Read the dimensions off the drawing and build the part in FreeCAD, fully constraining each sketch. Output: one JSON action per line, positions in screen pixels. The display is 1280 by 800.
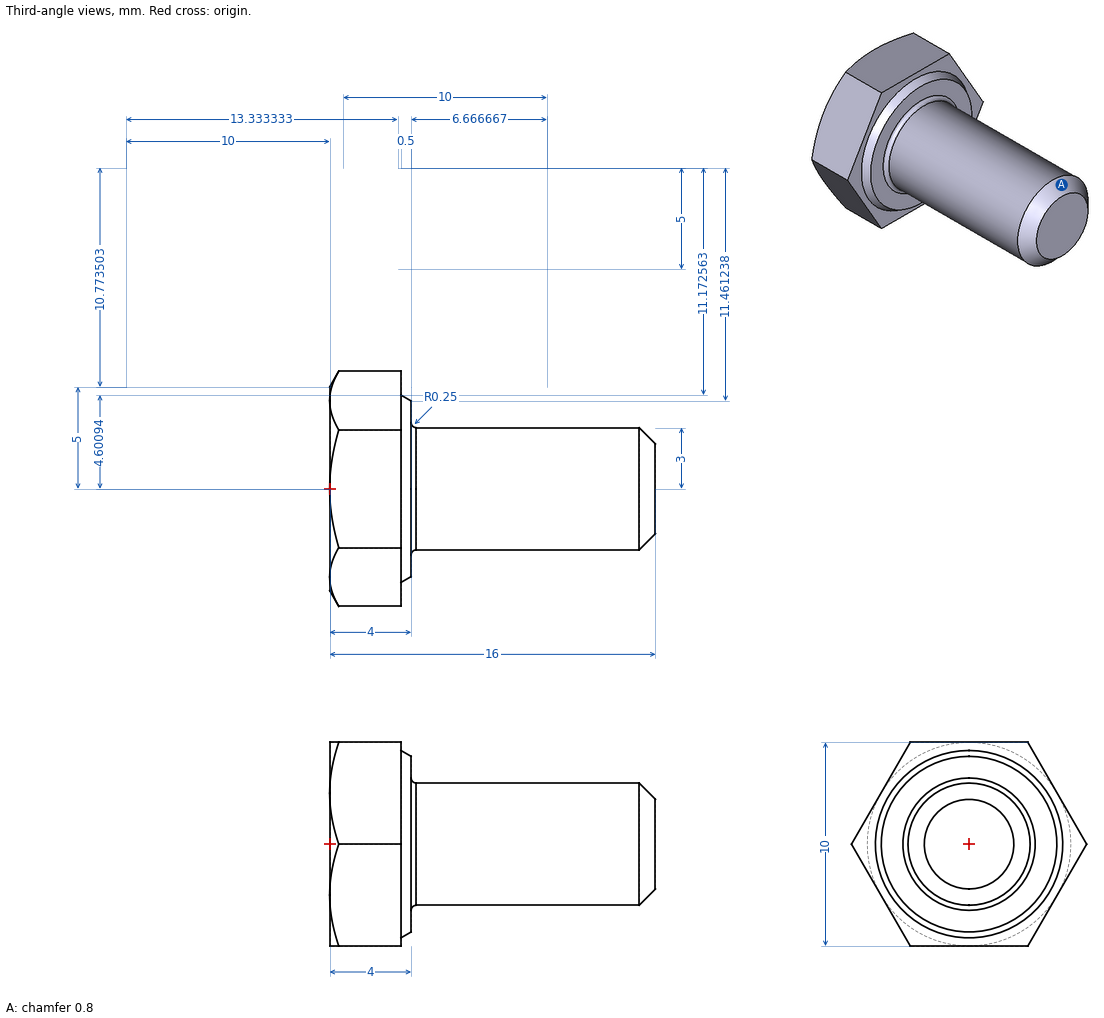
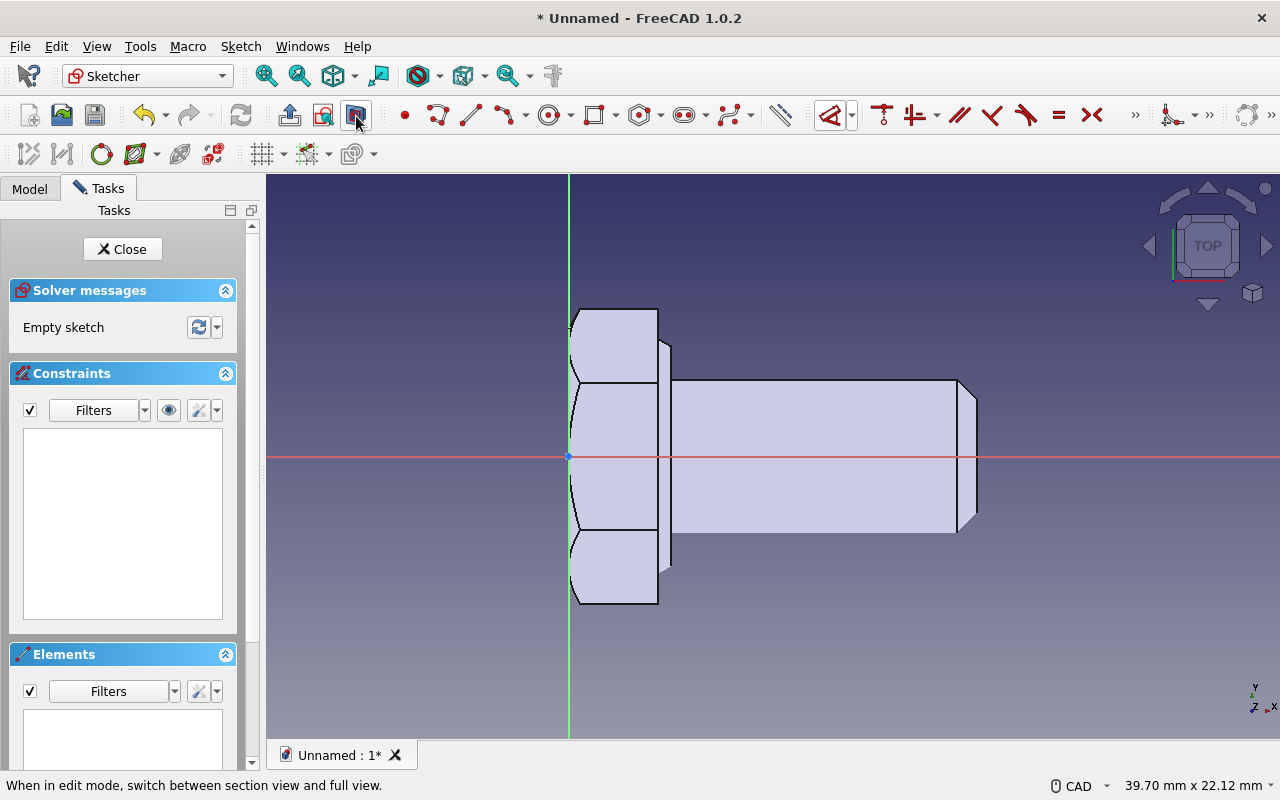
{"action": "scroll", "coordinate": [672, 373], "scroll_direction": "up", "scroll_amount": 15}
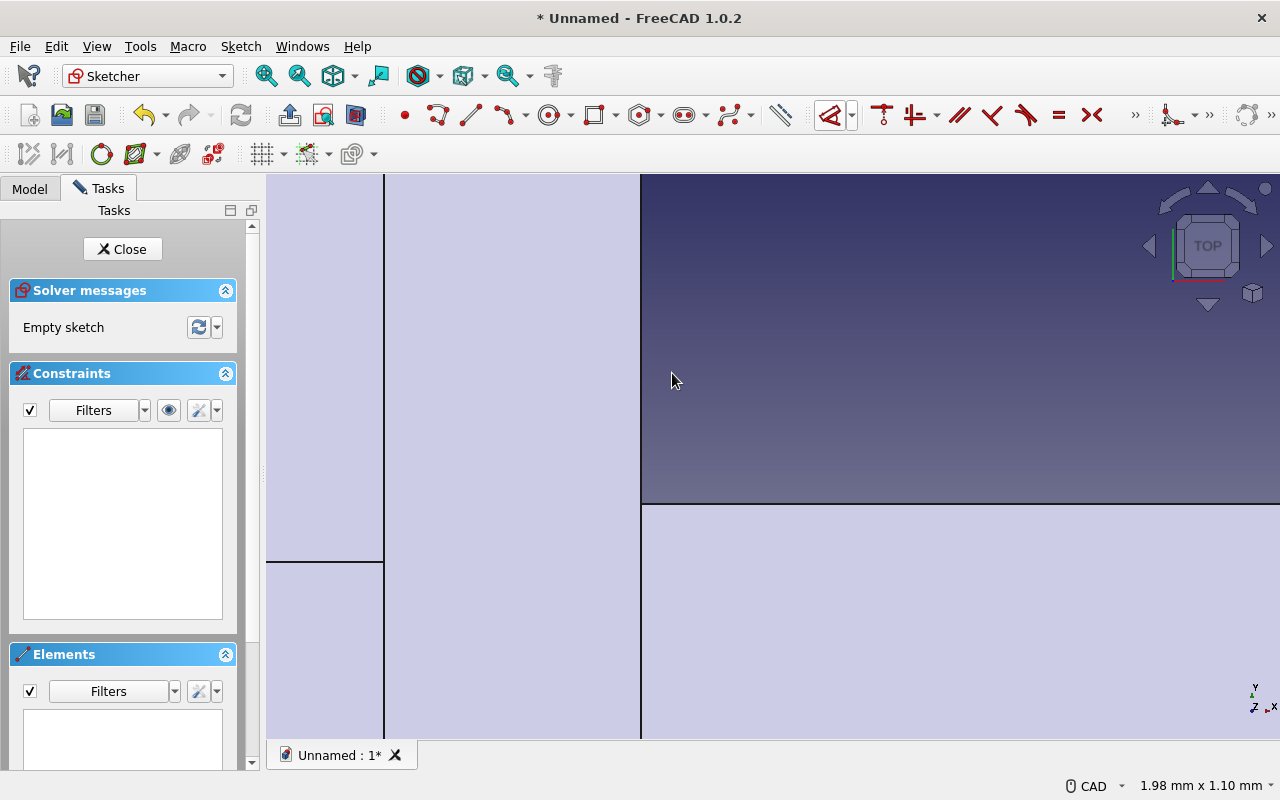
{"action": "scroll", "coordinate": [705, 431], "scroll_direction": "up", "scroll_amount": 5}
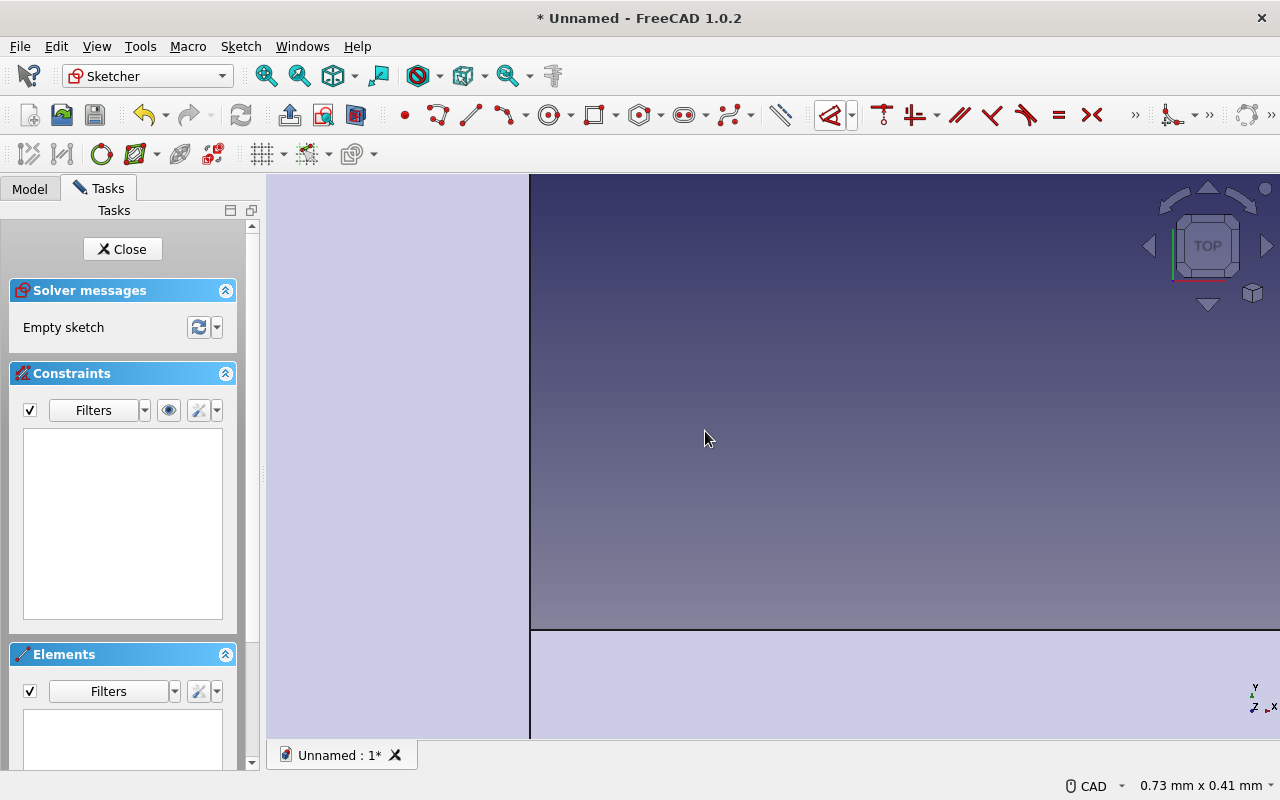
{"action": "left_click", "coordinate": [438, 116]}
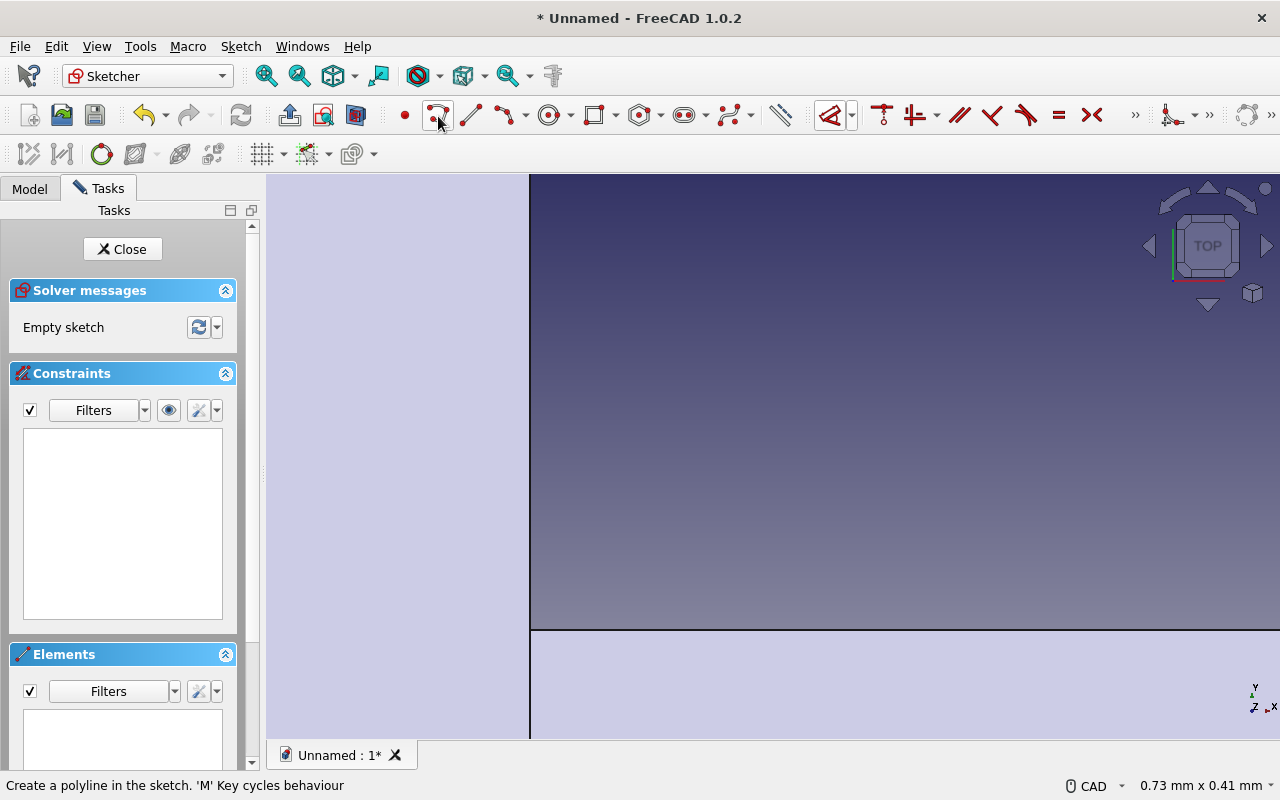
{"action": "left_click", "coordinate": [530, 281]}
{"action": "left_click", "coordinate": [530, 630]}
{"action": "left_click", "coordinate": [879, 630]}
{"action": "right_click", "coordinate": [879, 630]}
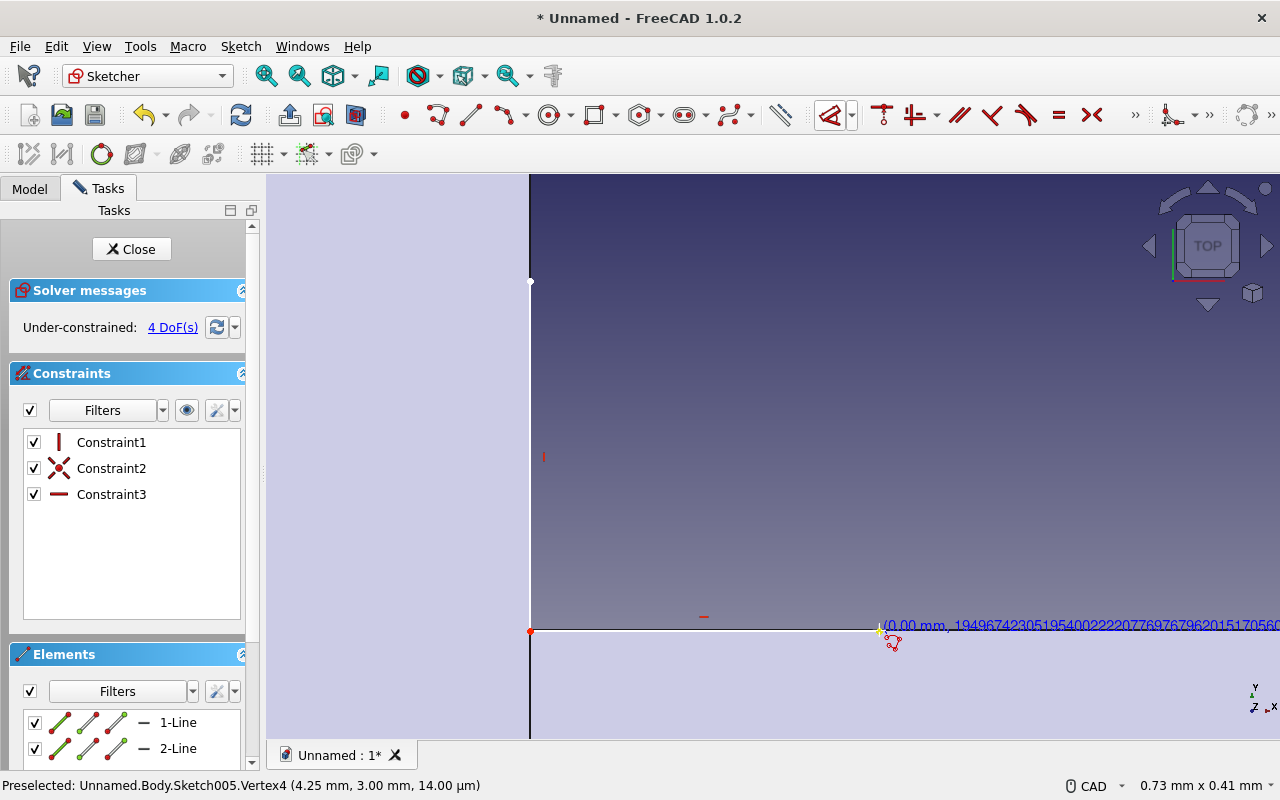
{"action": "left_click", "coordinate": [504, 116]}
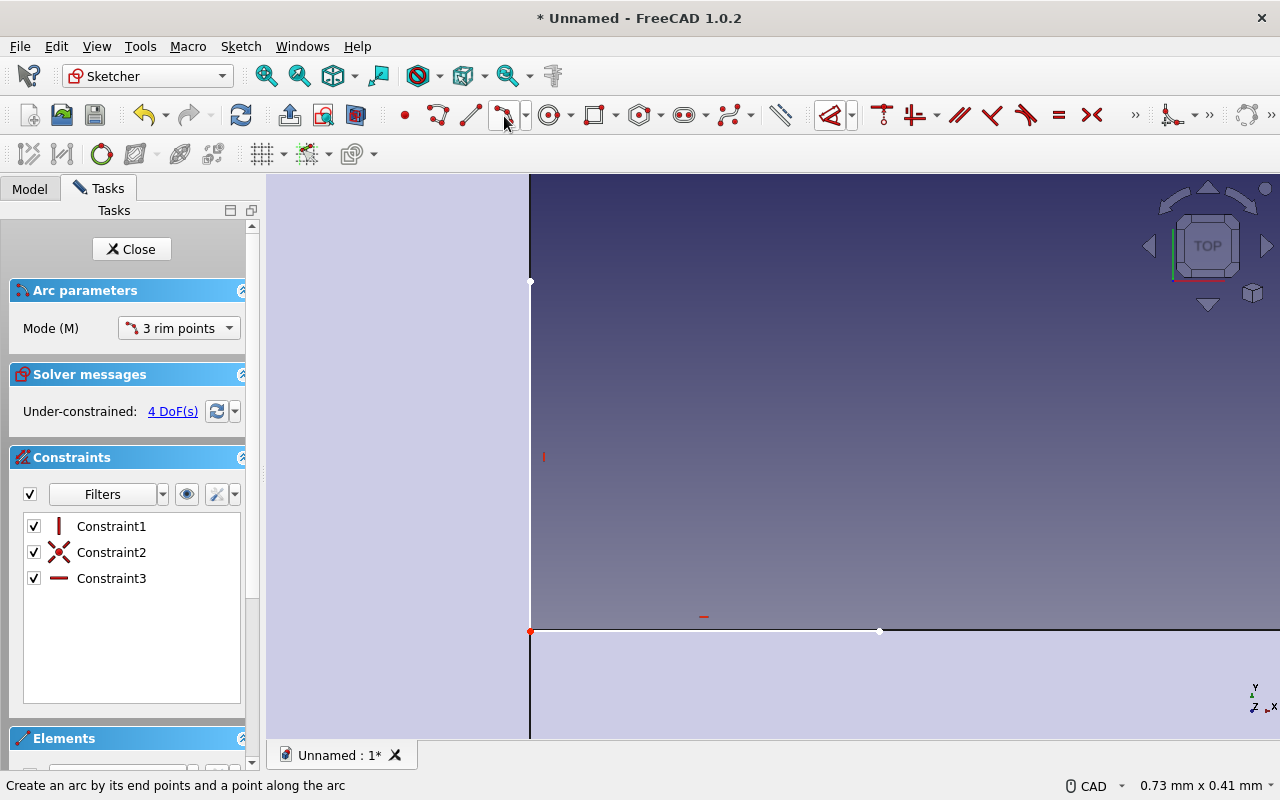
{"action": "left_click", "coordinate": [879, 631]}
{"action": "left_click", "coordinate": [530, 282]}
{"action": "left_click", "coordinate": [632, 528]}
{"action": "key", "text": "Escape"}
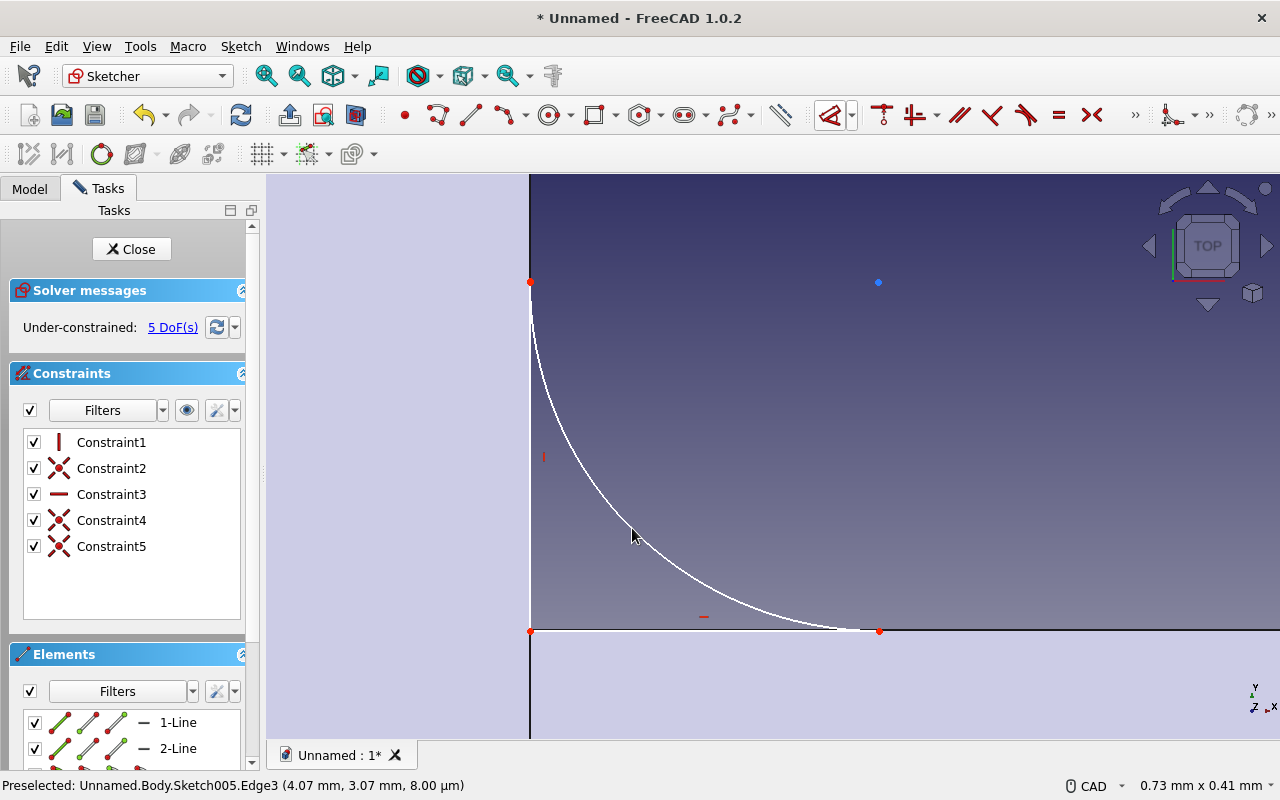
{"action": "left_click", "coordinate": [530, 387]}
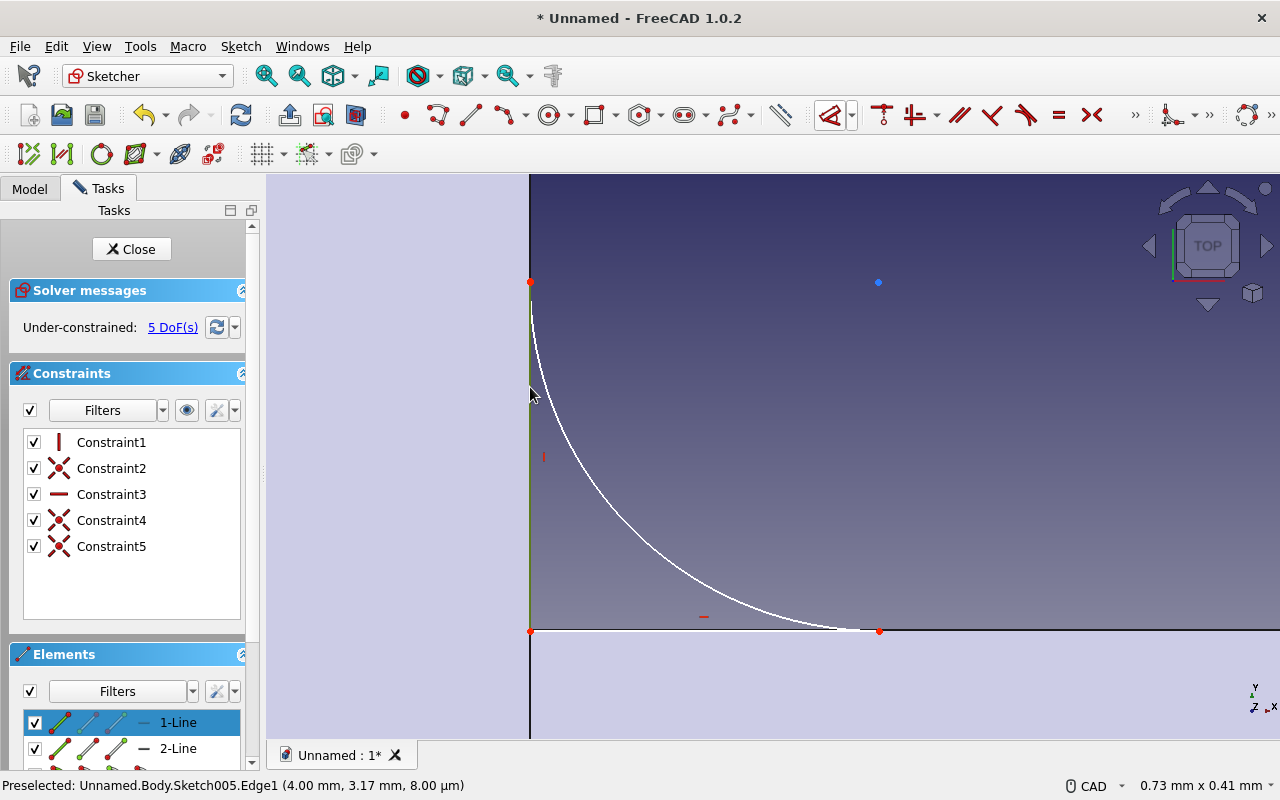
{"action": "left_click", "coordinate": [568, 441]}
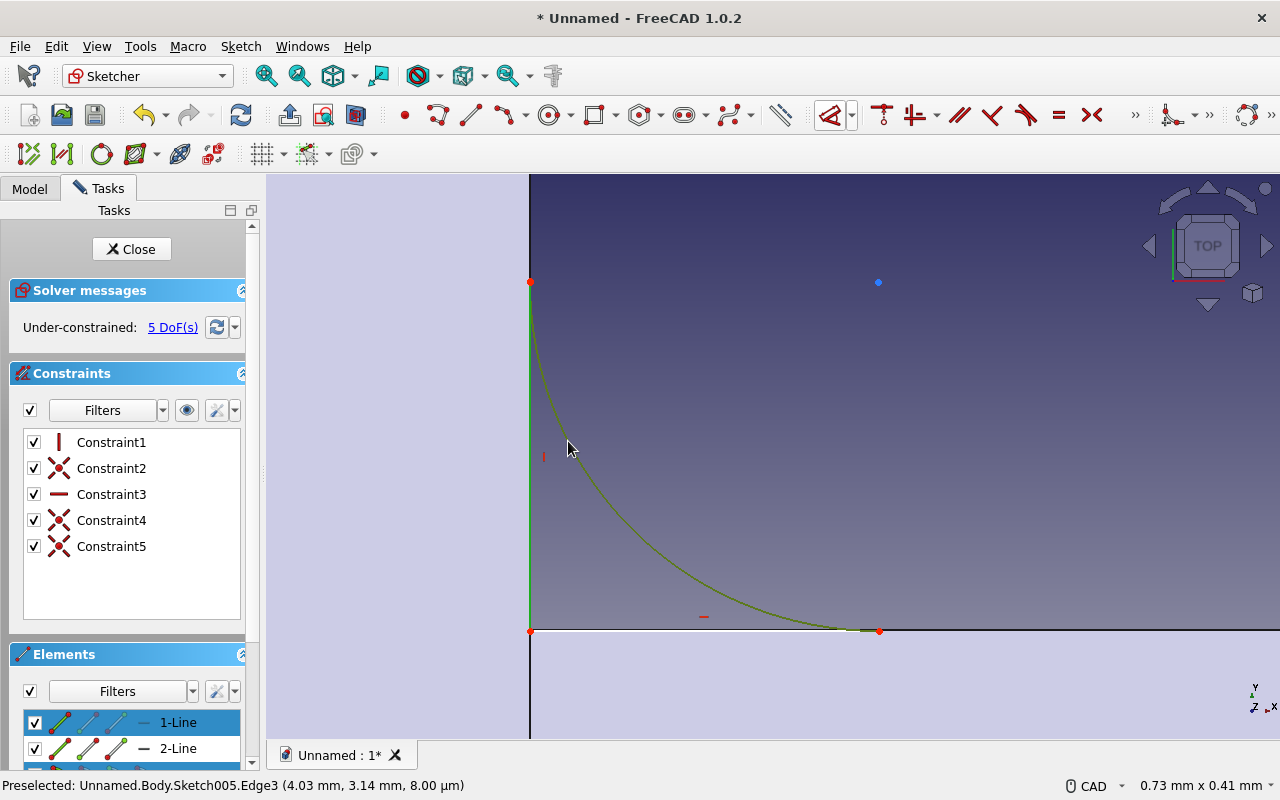
{"action": "left_click", "coordinate": [1026, 116]}